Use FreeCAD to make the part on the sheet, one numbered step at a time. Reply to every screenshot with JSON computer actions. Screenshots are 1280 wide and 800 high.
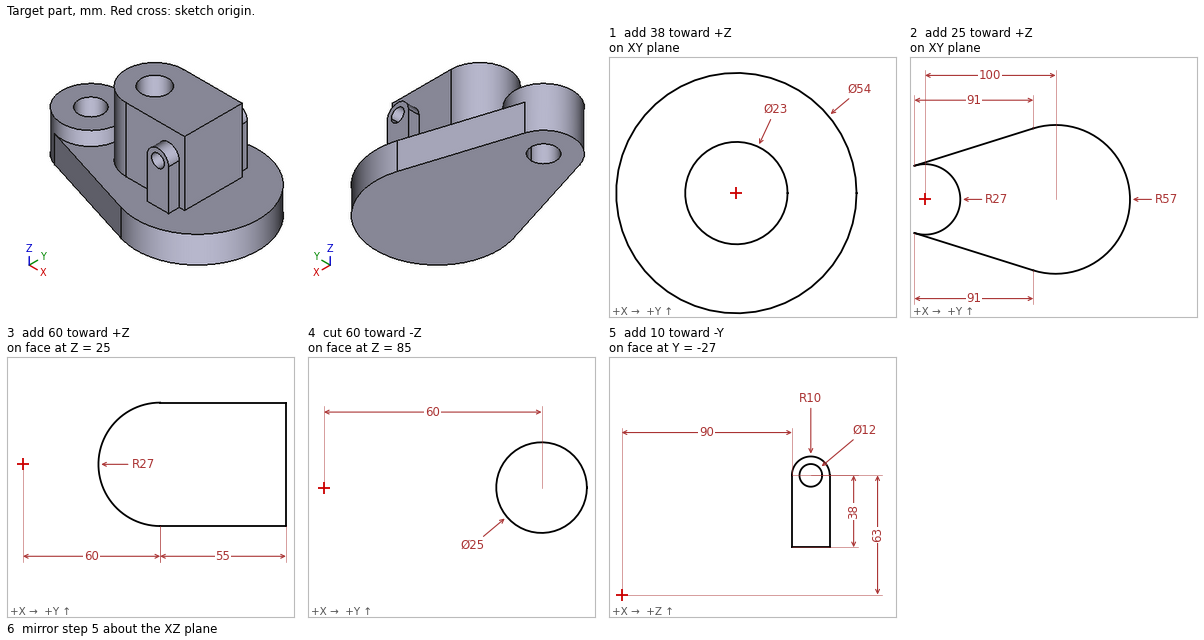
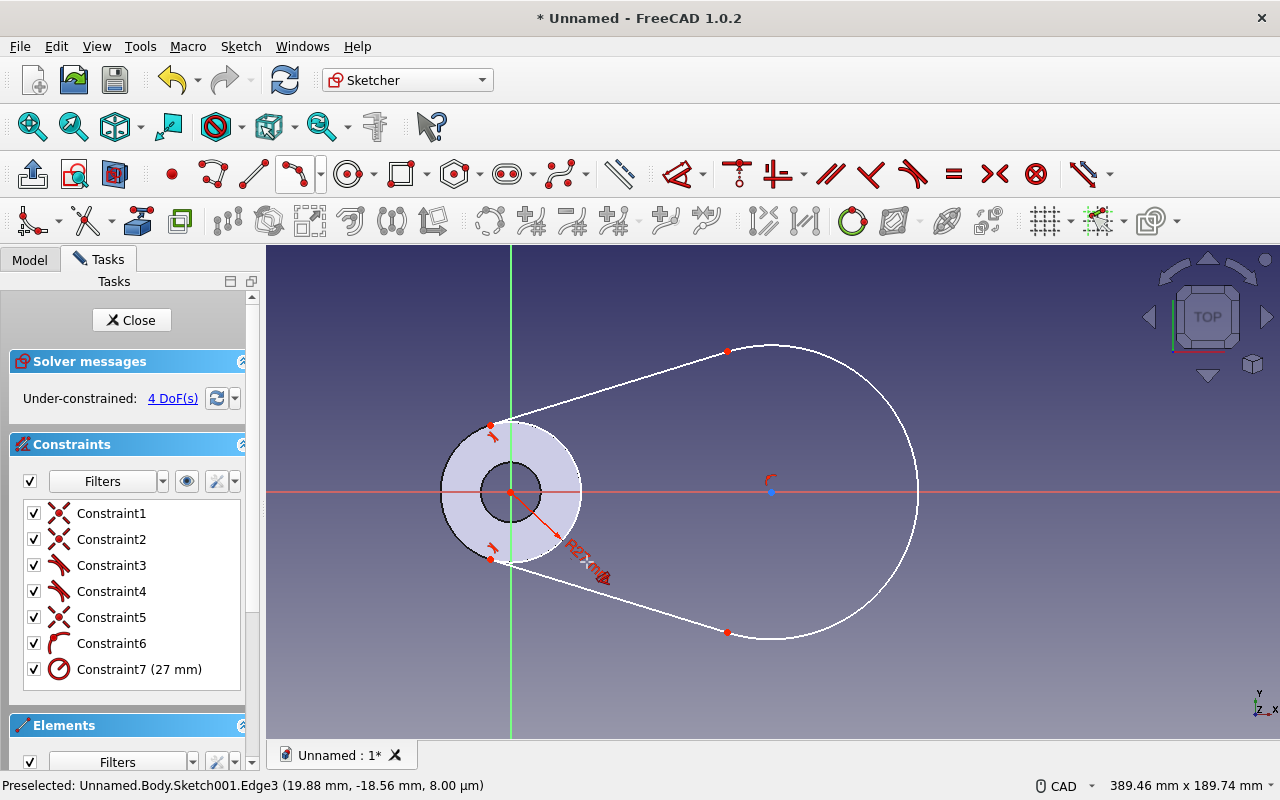
{"action": "left_click", "coordinate": [879, 593]}
{"action": "left_click", "coordinate": [902, 615]}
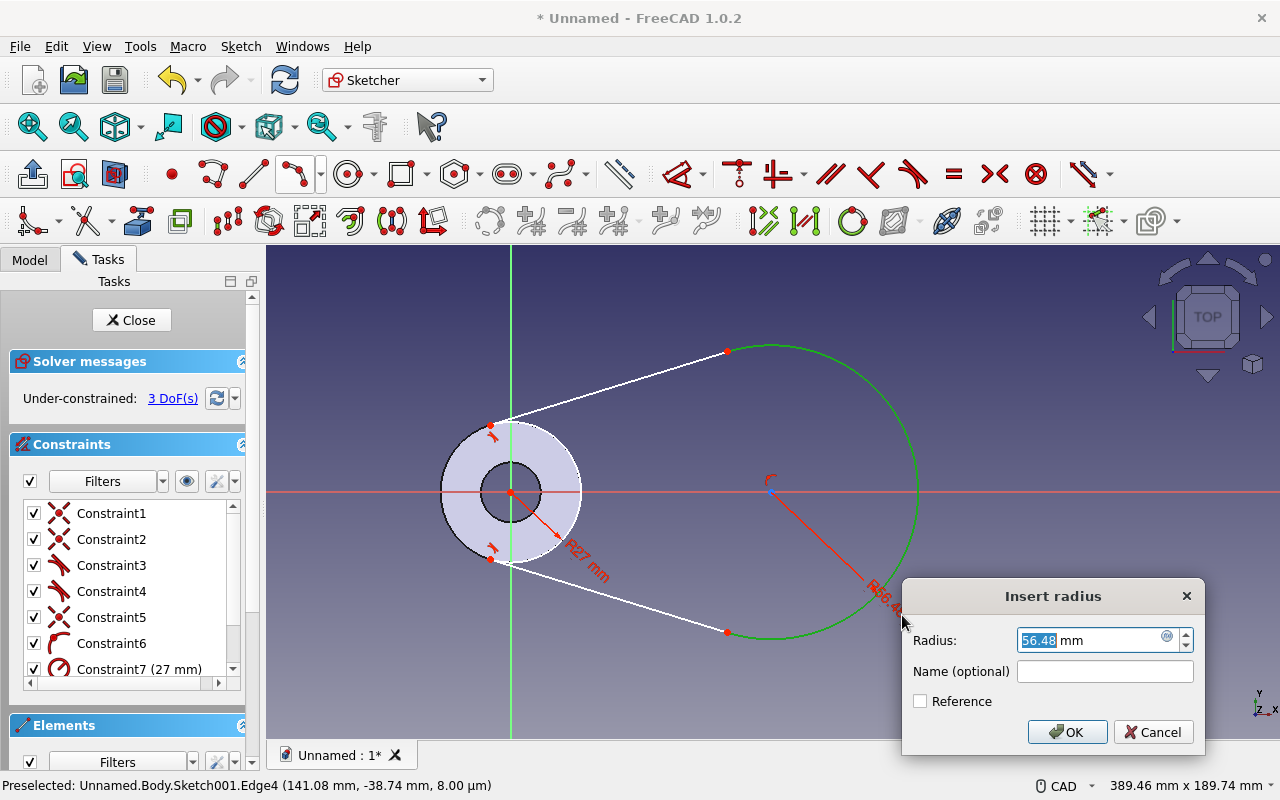
{"action": "type", "text": "57"}
{"action": "key", "text": "Return"}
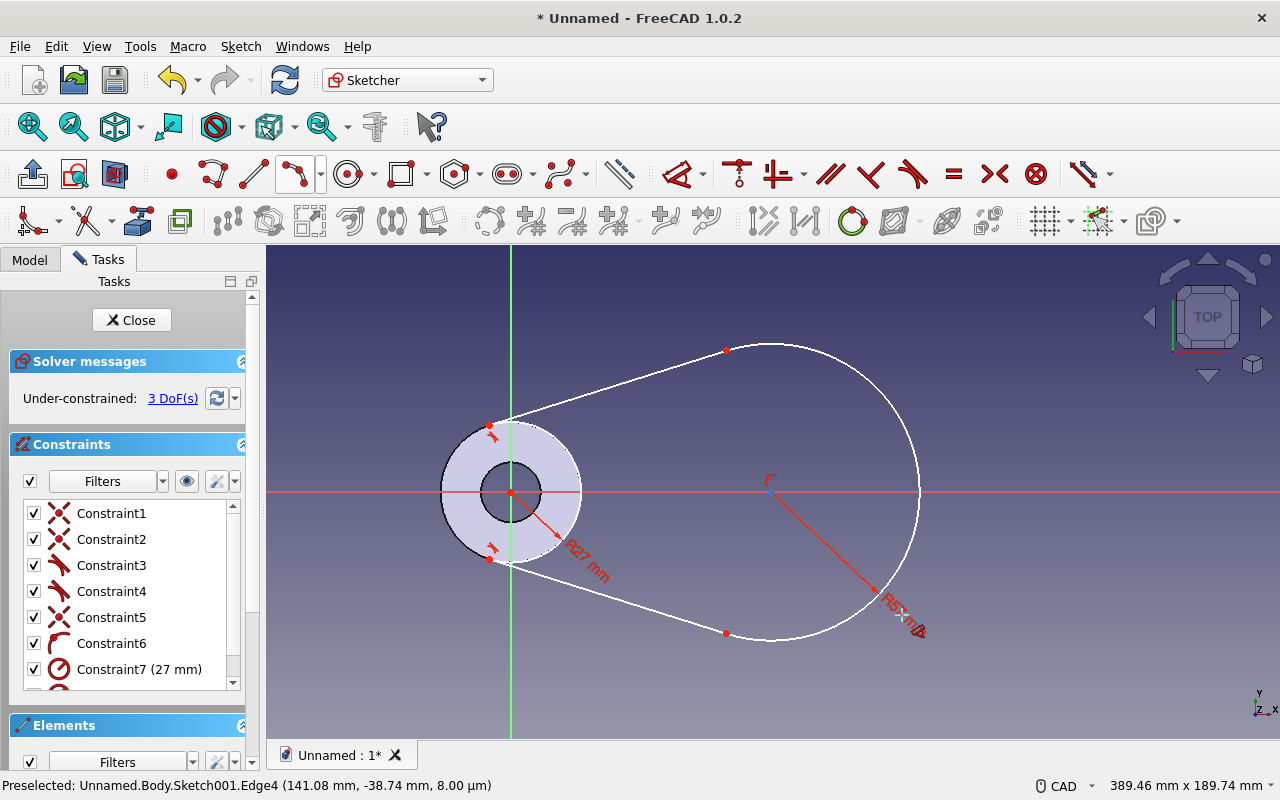
{"action": "left_click", "coordinate": [656, 373]}
{"action": "left_click", "coordinate": [608, 317]}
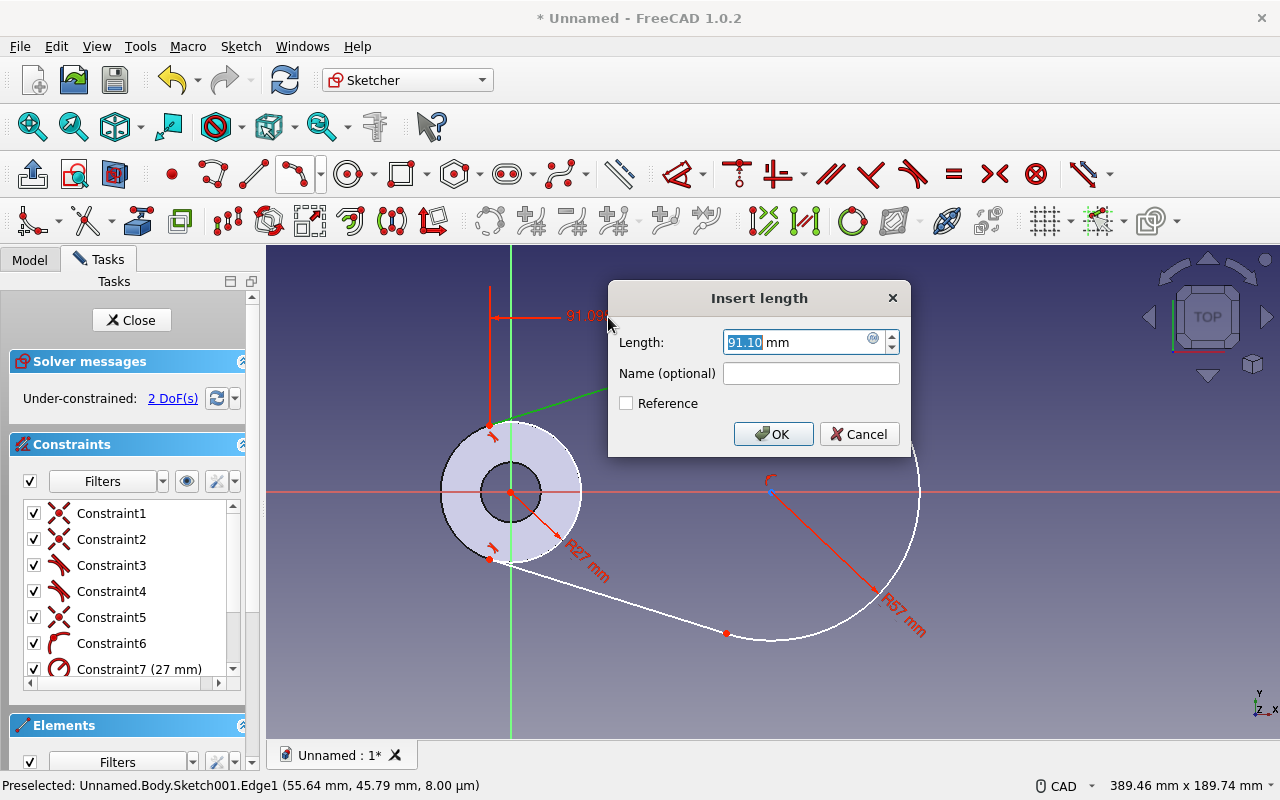
{"action": "type", "text": "91"}
{"action": "key", "text": "Return"}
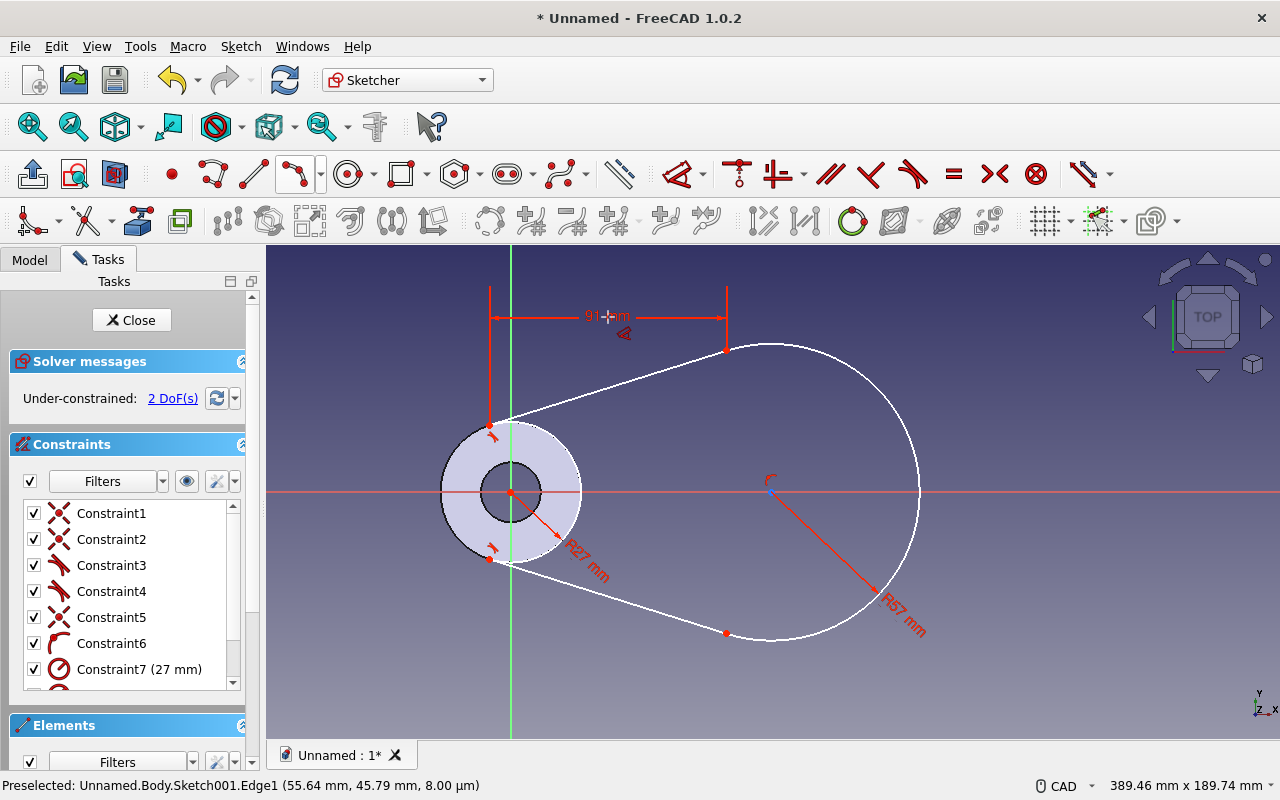
{"action": "left_click", "coordinate": [561, 582]}
{"action": "left_click", "coordinate": [608, 668]}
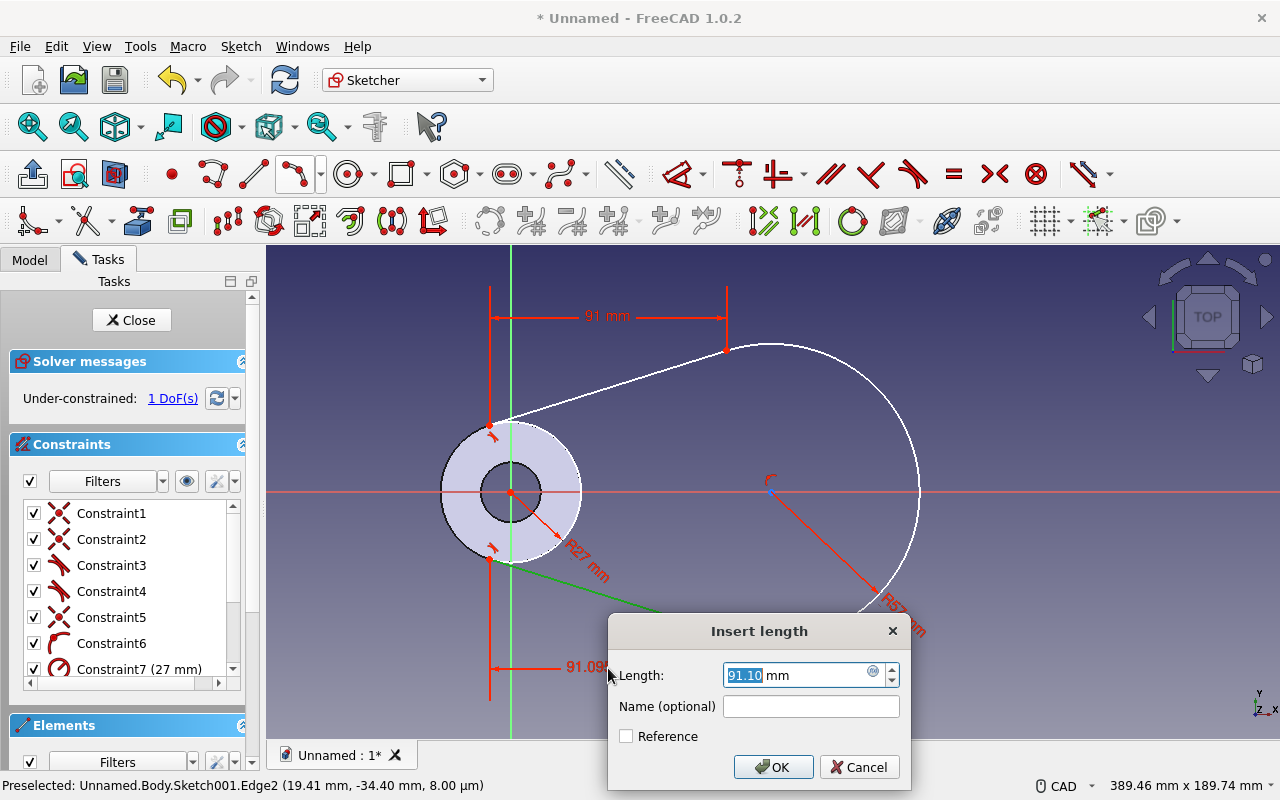
{"action": "type", "text": "91"}
{"action": "key", "text": "Return"}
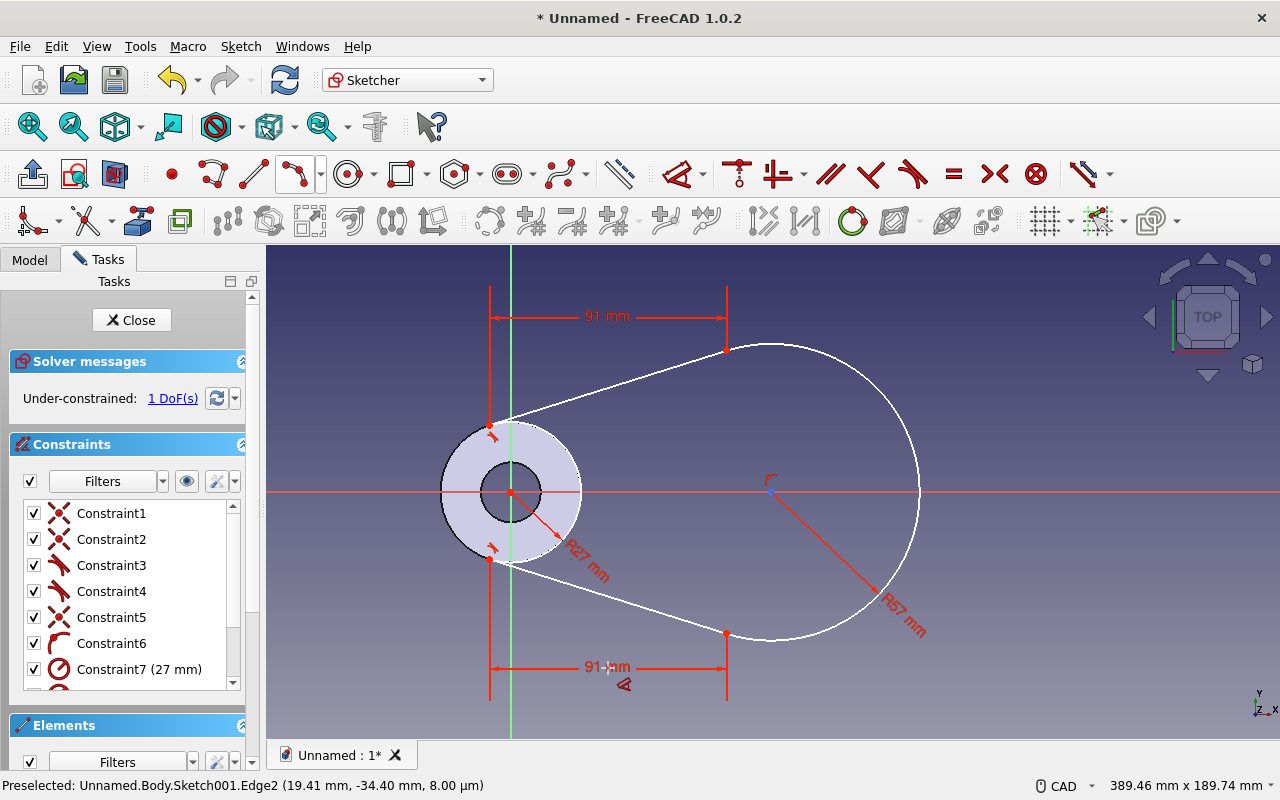
{"action": "left_click", "coordinate": [771, 492]}
{"action": "left_click", "coordinate": [641, 526]}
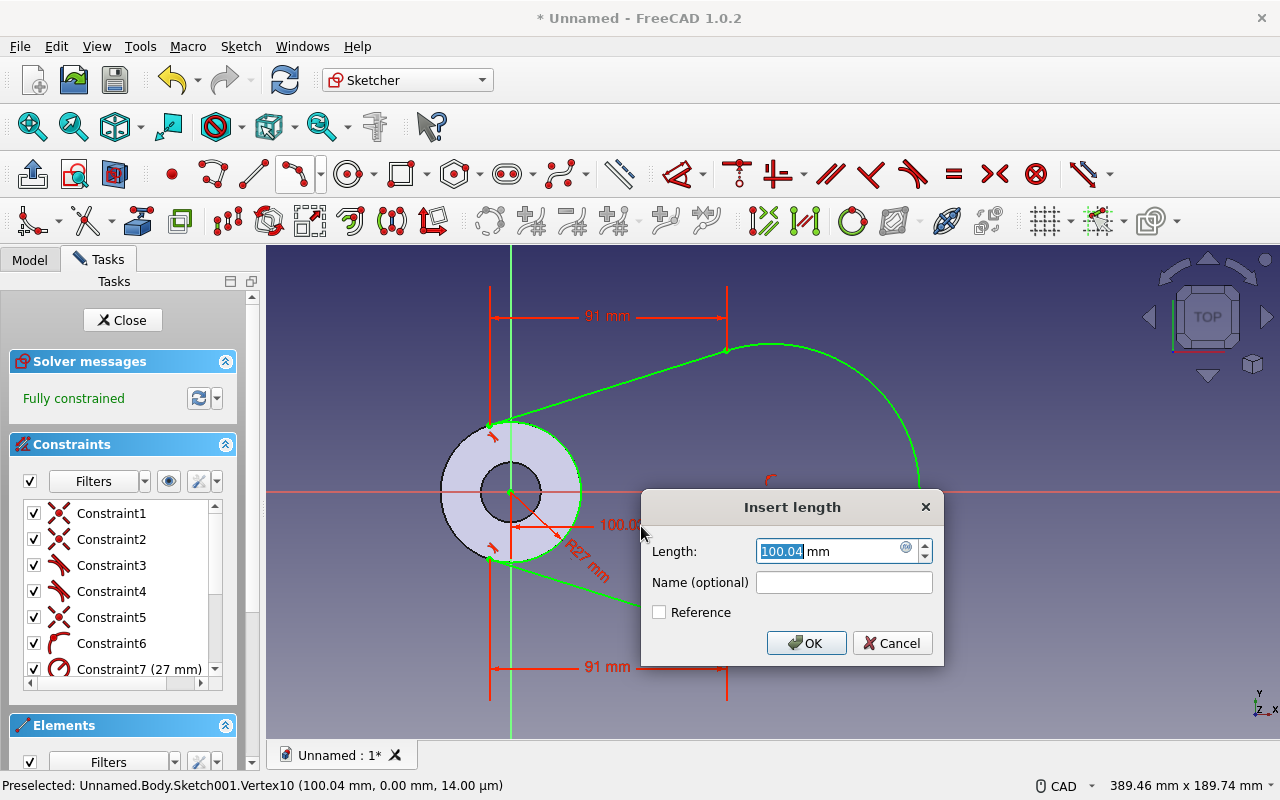
{"action": "type", "text": "100"}
{"action": "key", "text": "Return"}
{"action": "key", "text": "Escape"}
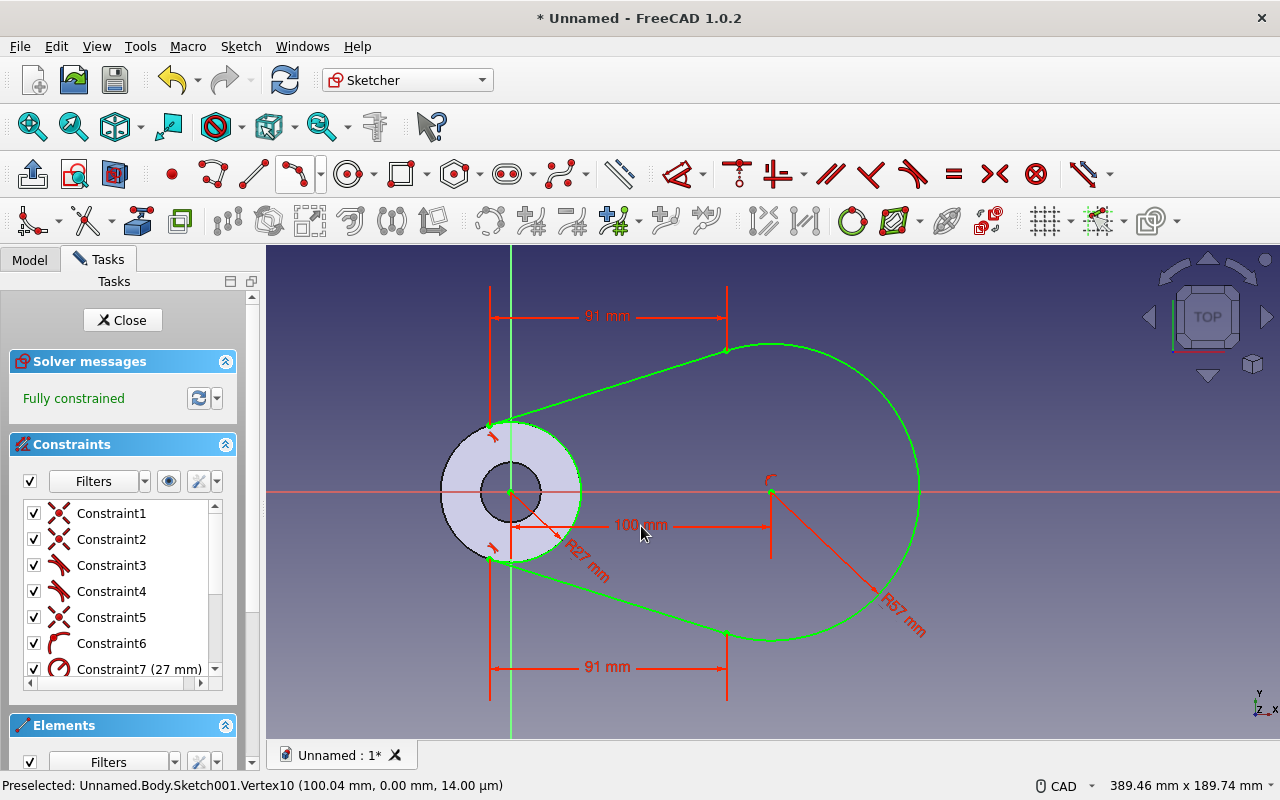
{"action": "left_click", "coordinate": [123, 320]}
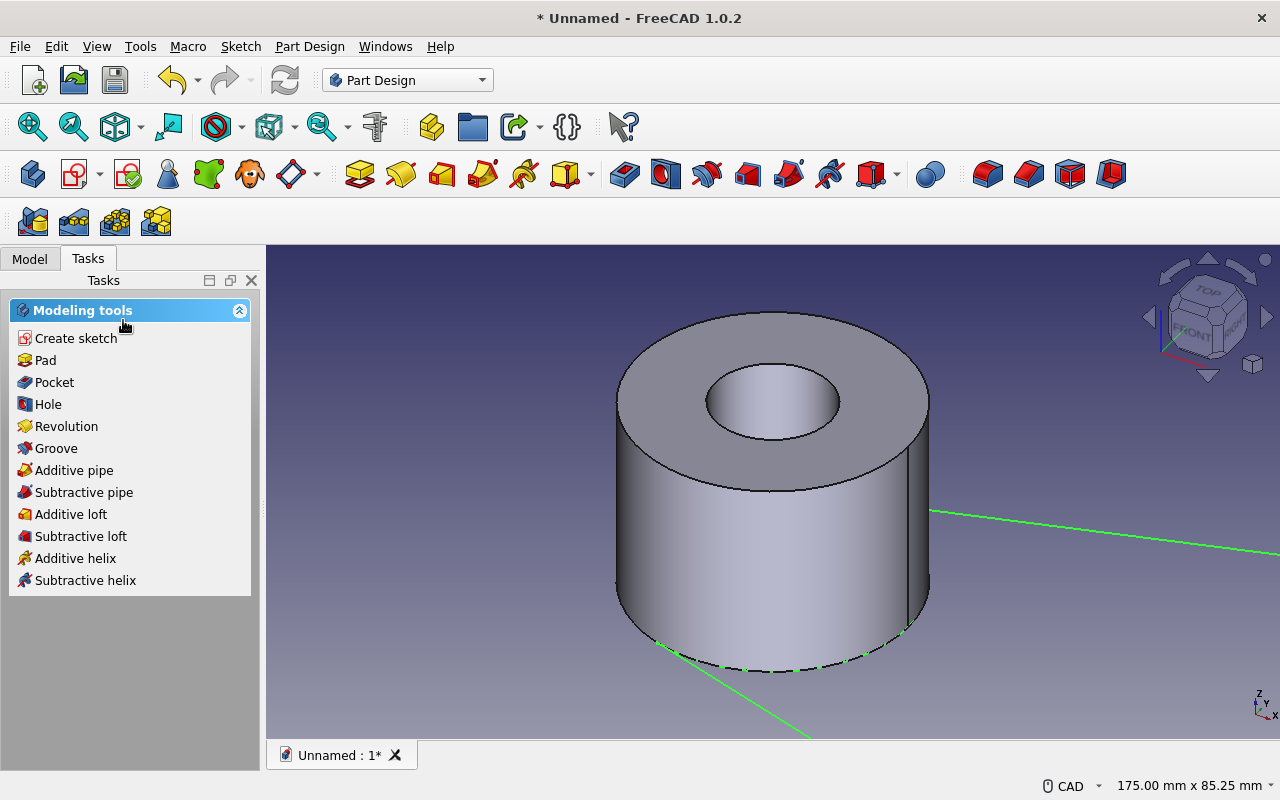
{"action": "left_click", "coordinate": [360, 174]}